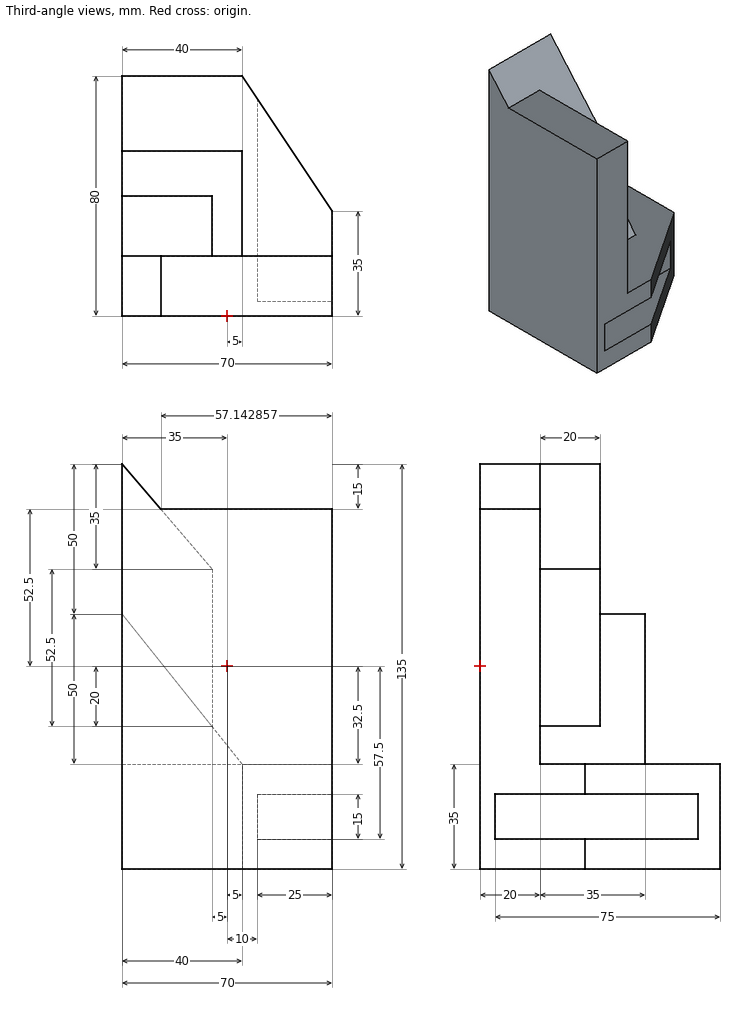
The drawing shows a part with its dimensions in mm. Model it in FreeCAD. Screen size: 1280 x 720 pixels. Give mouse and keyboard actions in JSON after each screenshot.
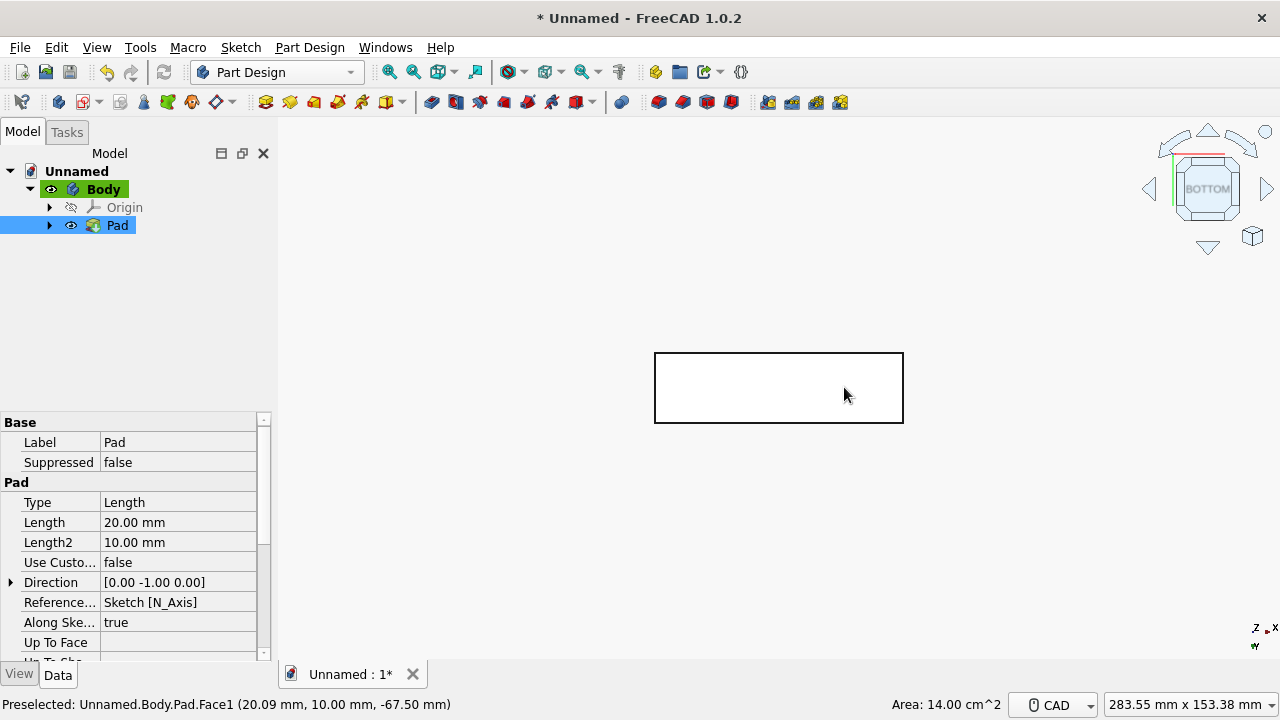
{"action": "left_click", "coordinate": [84, 102]}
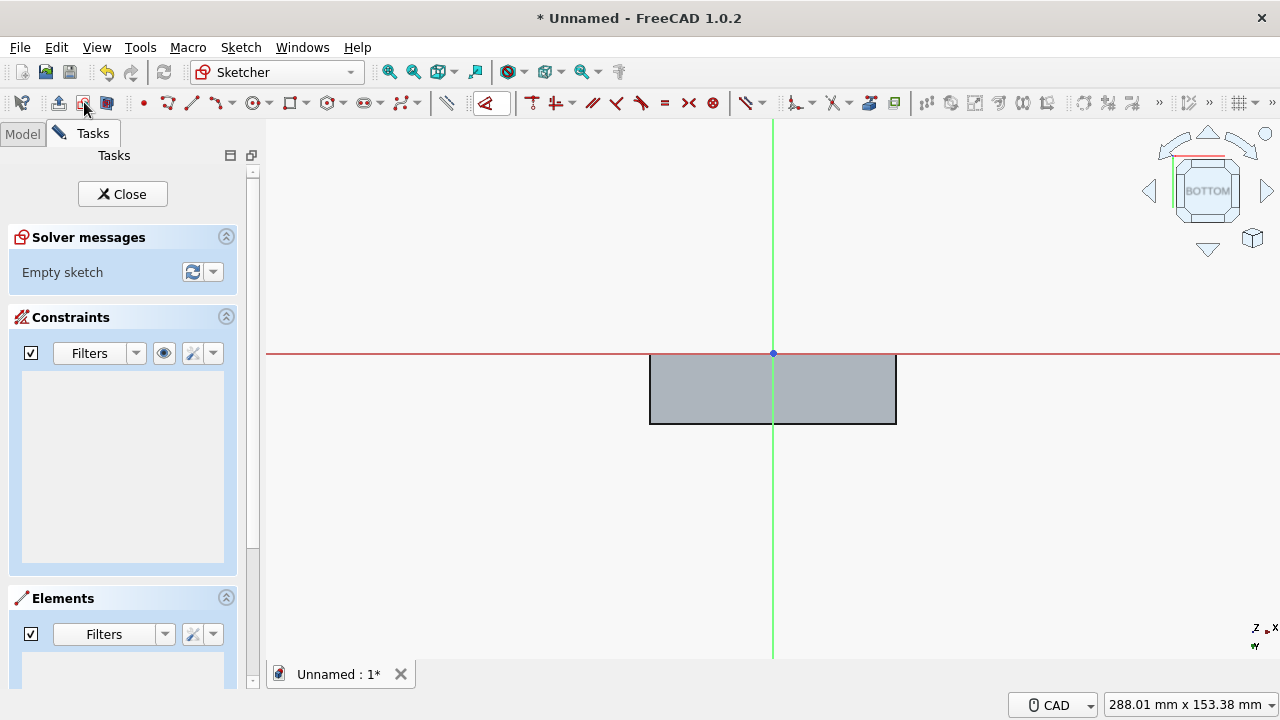
{"action": "scroll", "coordinate": [395, 147], "scroll_direction": "down", "scroll_amount": 1}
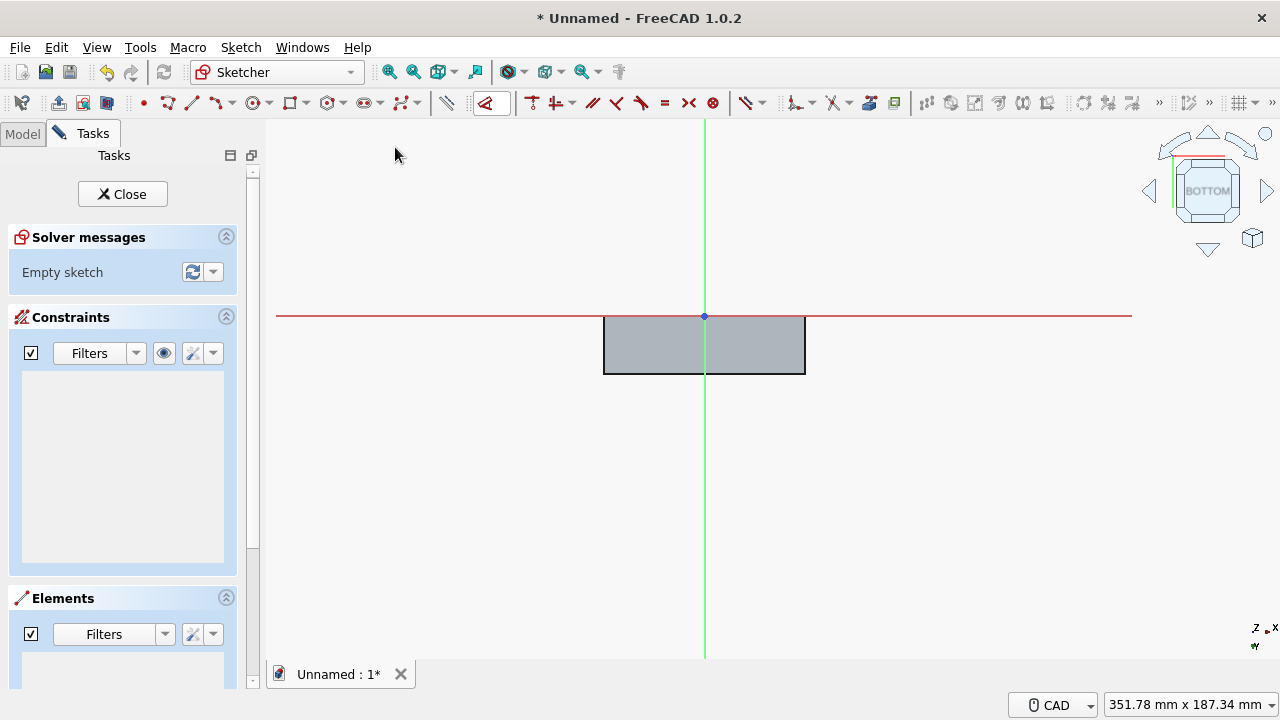
{"action": "scroll", "coordinate": [705, 518], "scroll_direction": "up", "scroll_amount": 2}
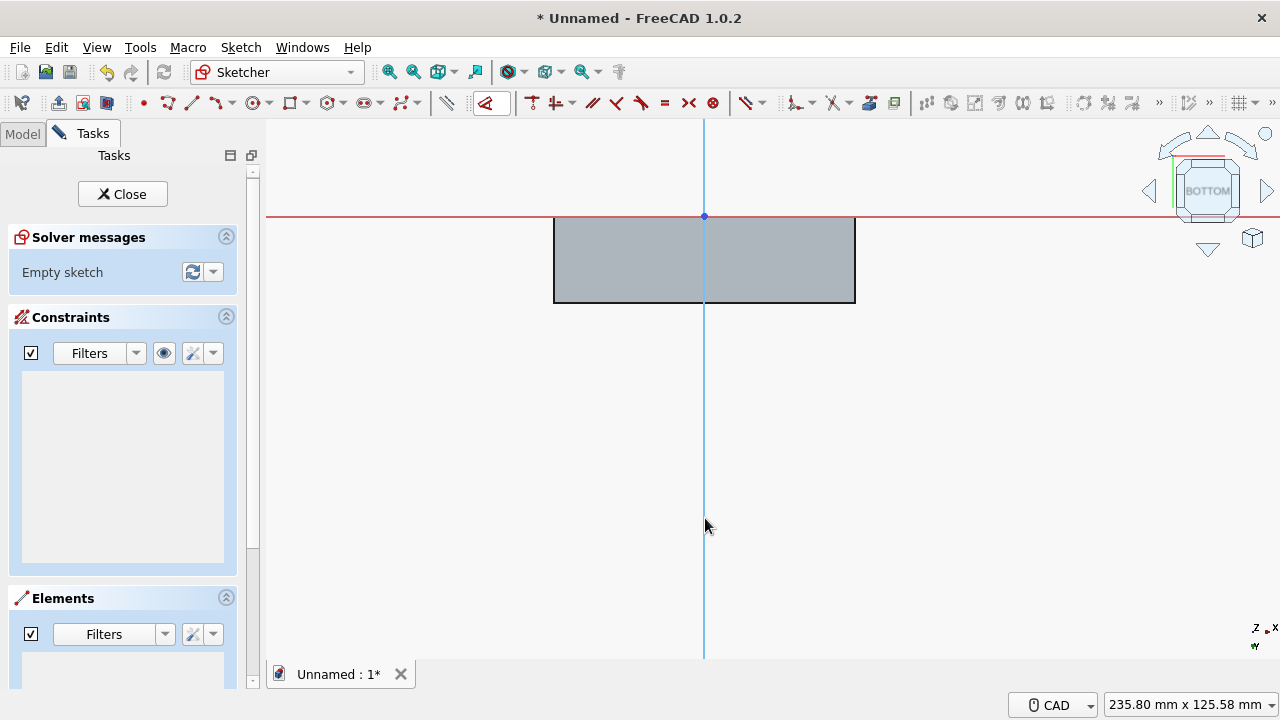
{"action": "left_click", "coordinate": [168, 104]}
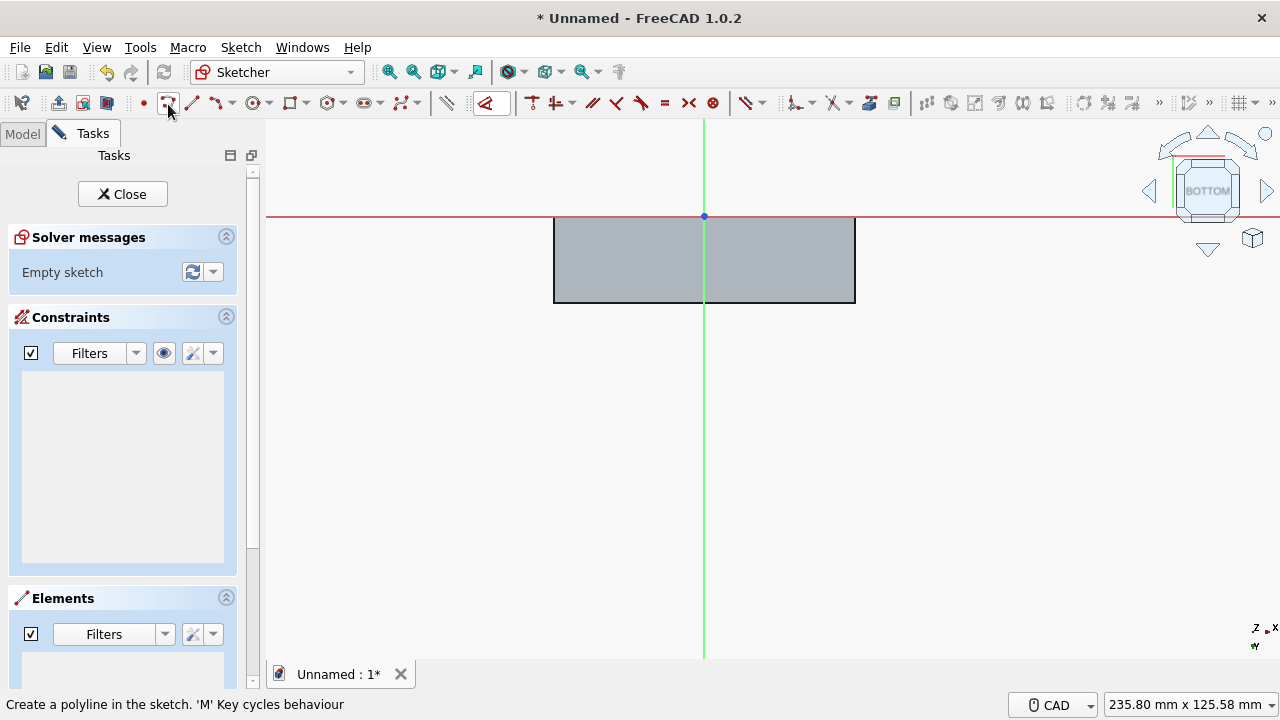
{"action": "left_click", "coordinate": [554, 217]}
{"action": "left_click", "coordinate": [554, 561]}
{"action": "left_click", "coordinate": [726, 561]}
{"action": "left_click", "coordinate": [855, 367]}
{"action": "left_click", "coordinate": [855, 226]}
{"action": "left_click", "coordinate": [554, 217]}
{"action": "key", "text": "Escape"}
{"action": "key", "text": "Escape"}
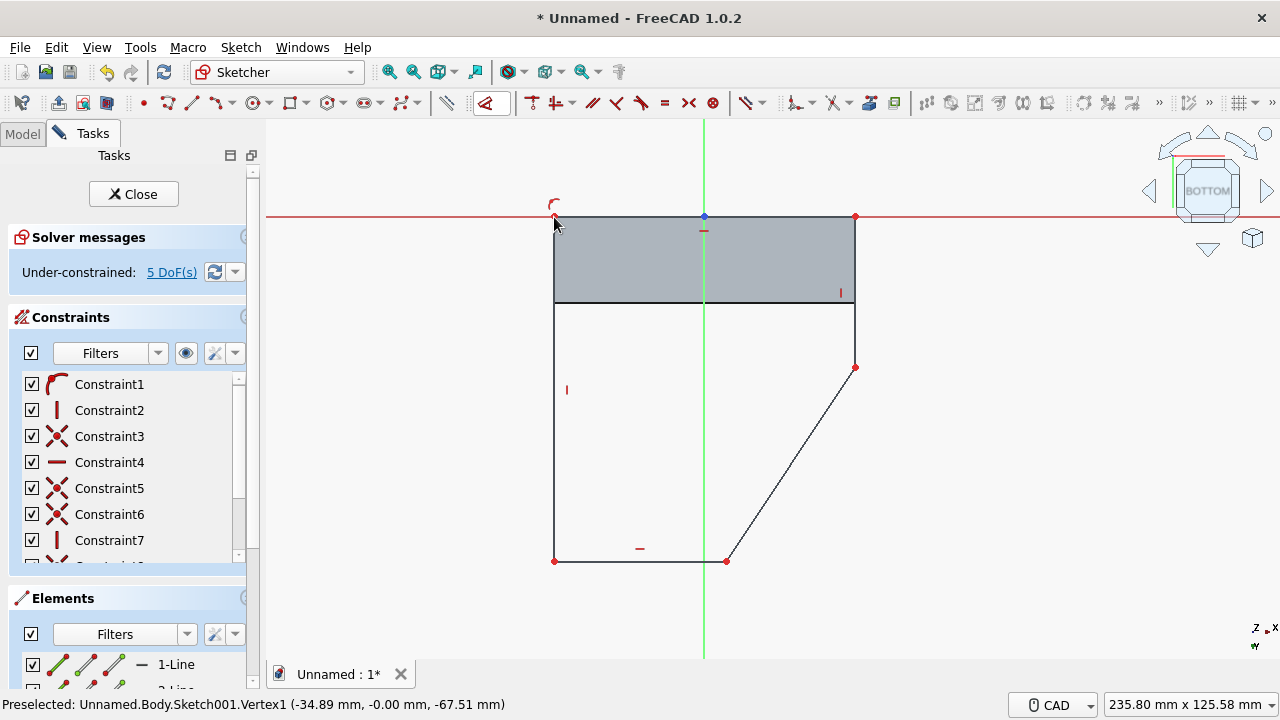
{"action": "left_click", "coordinate": [554, 320]}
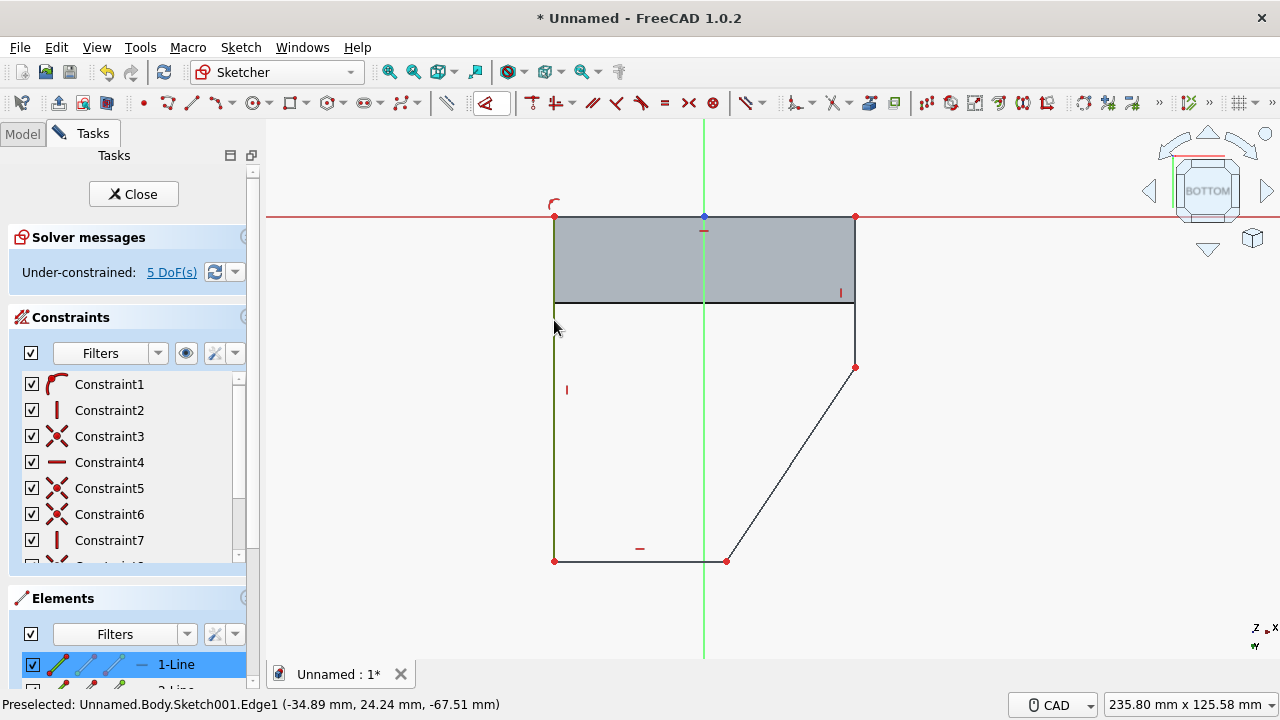
{"action": "key", "text": "i"}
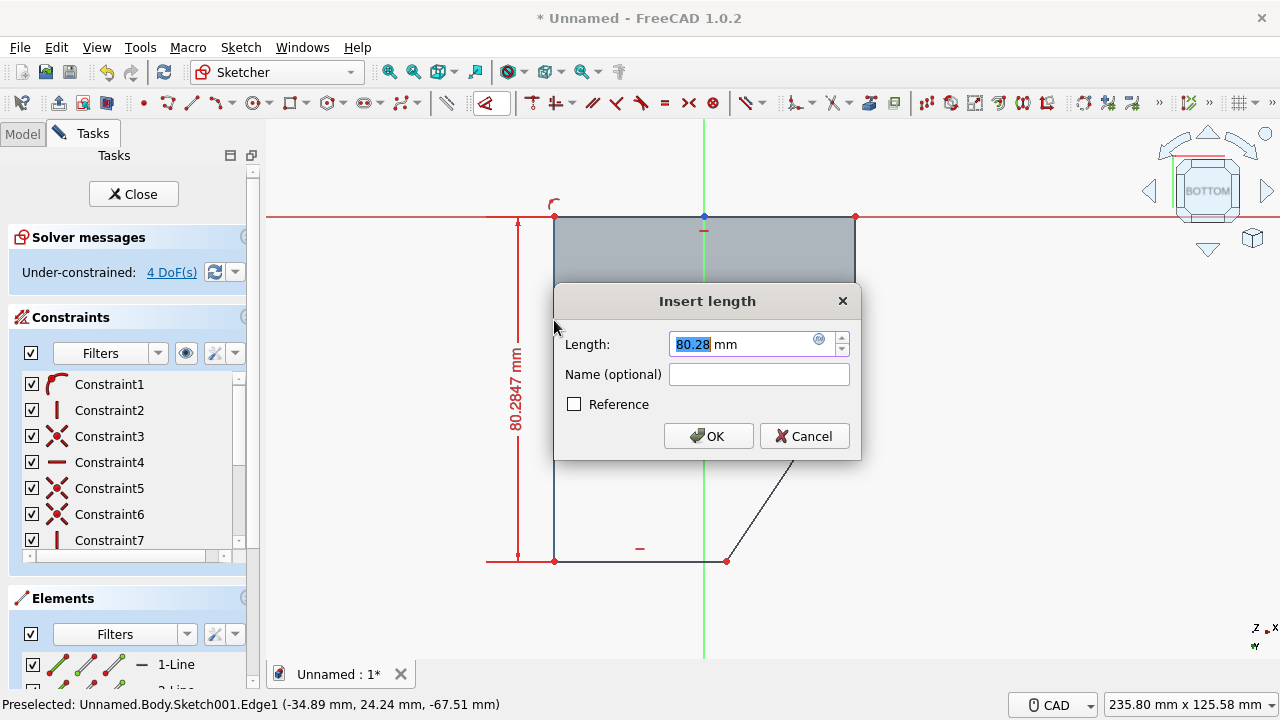
{"action": "type", "text": "80"}
{"action": "key", "text": "Return"}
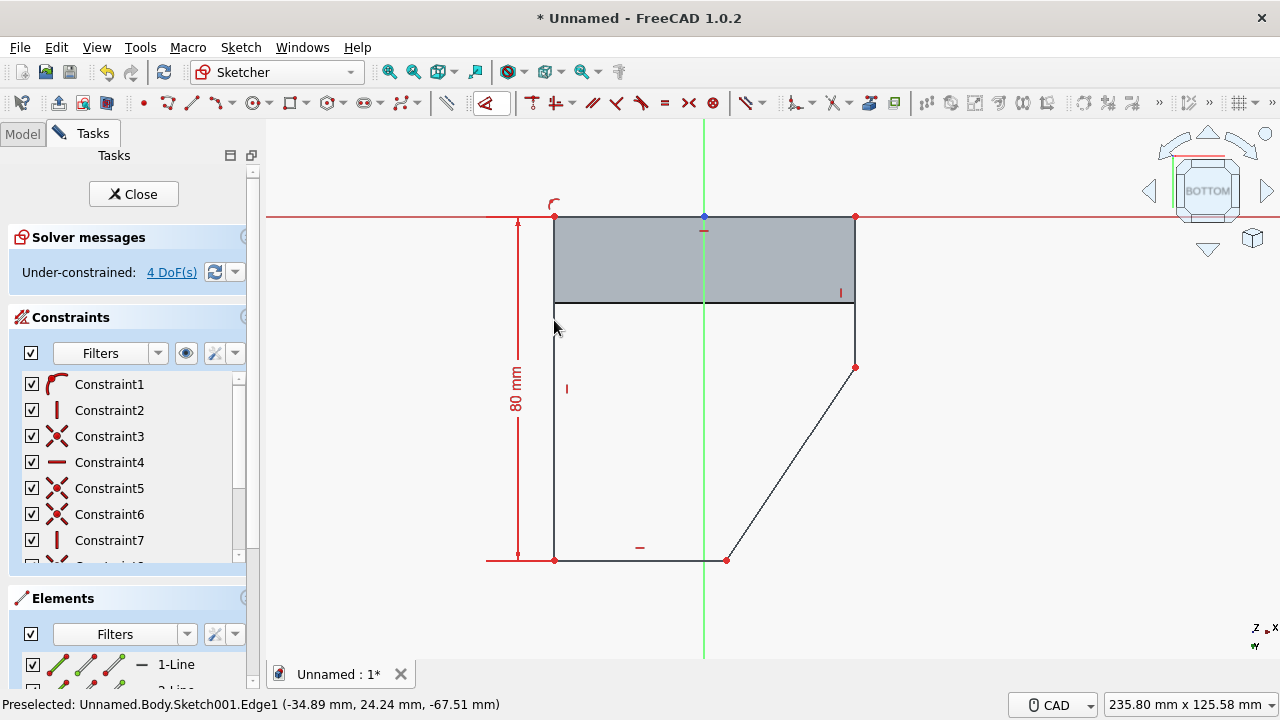
{"action": "left_click", "coordinate": [606, 561]}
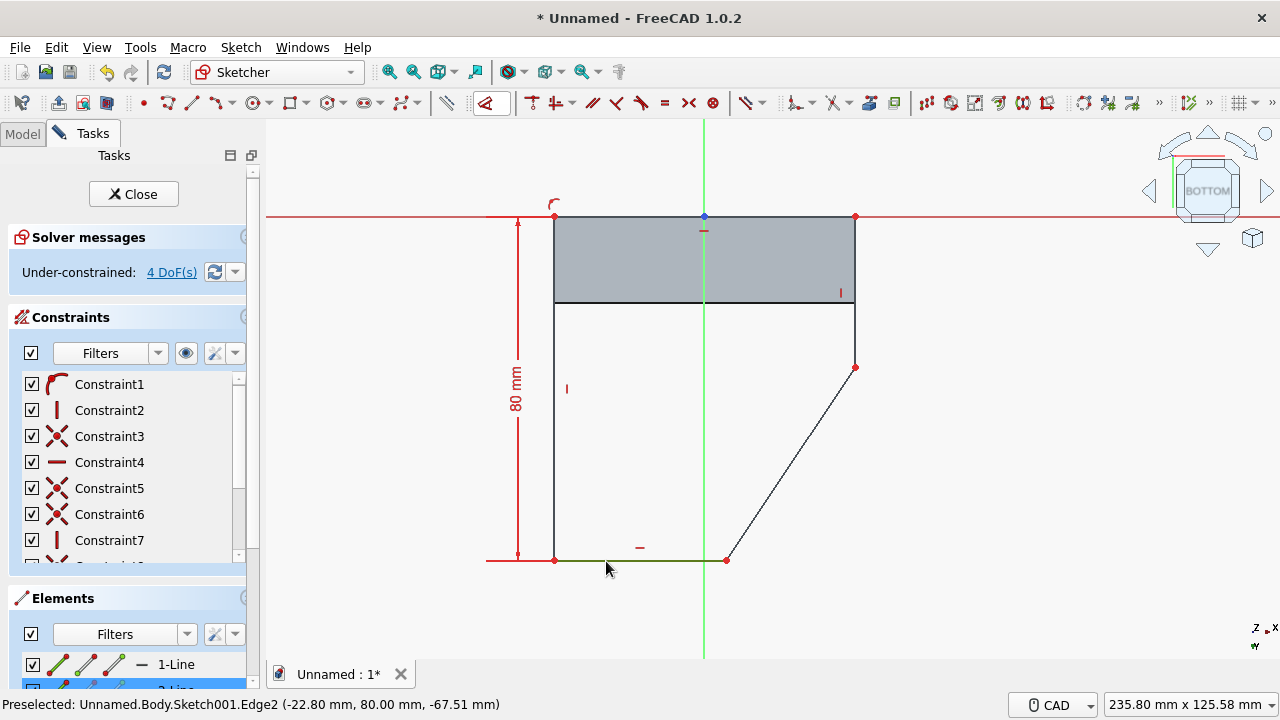
{"action": "left_click", "coordinate": [504, 104]}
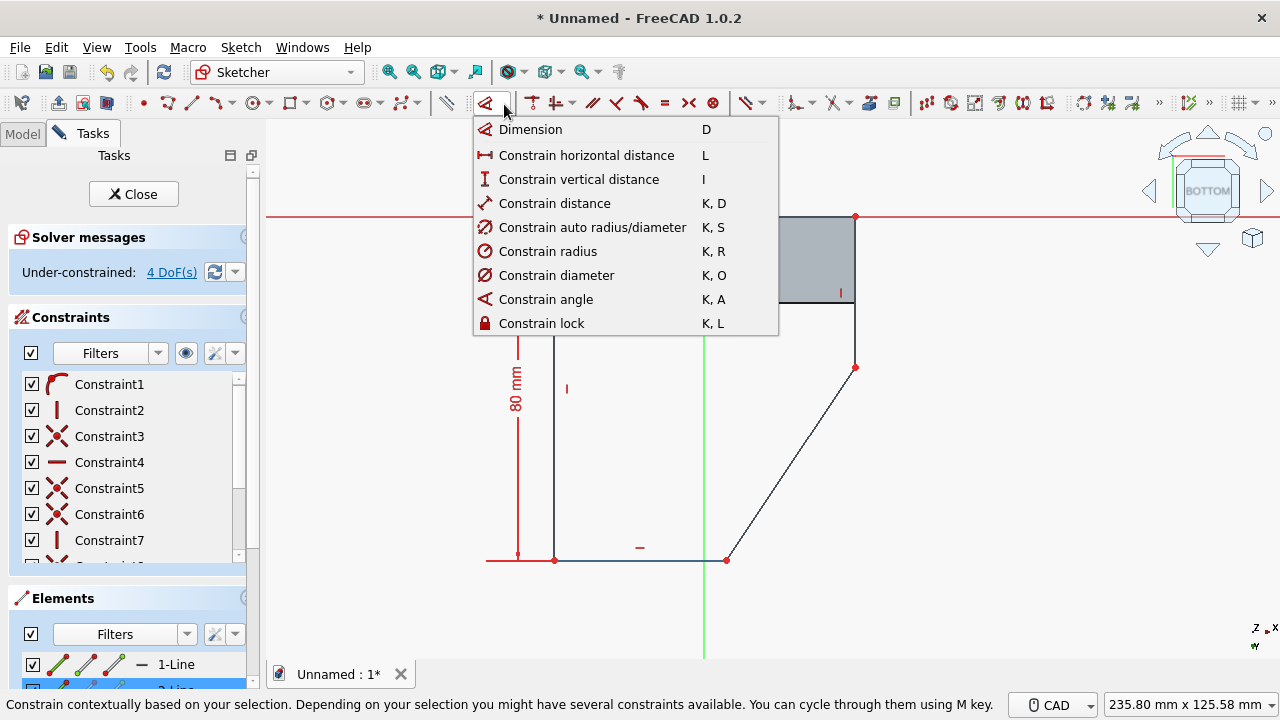
{"action": "left_click", "coordinate": [626, 155]}